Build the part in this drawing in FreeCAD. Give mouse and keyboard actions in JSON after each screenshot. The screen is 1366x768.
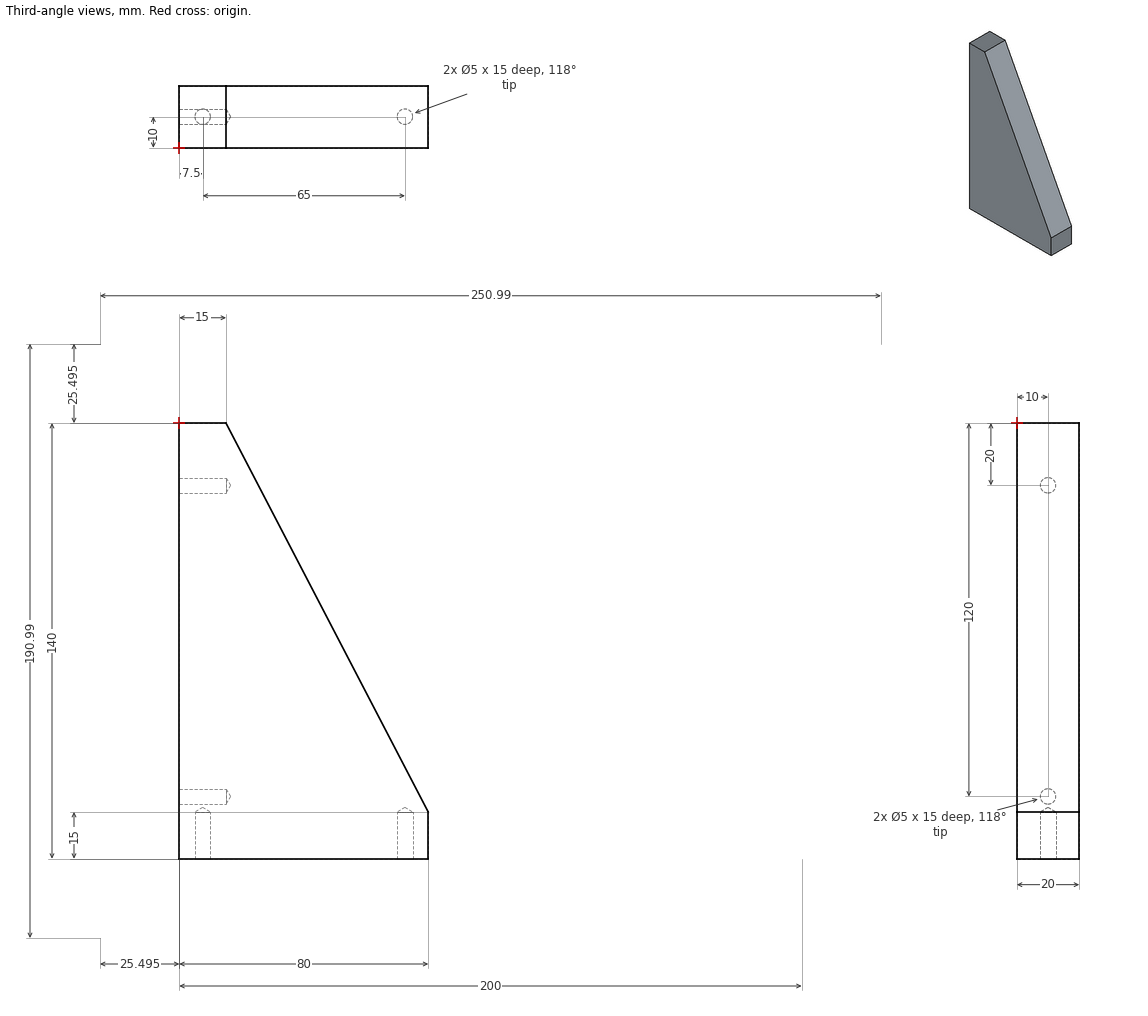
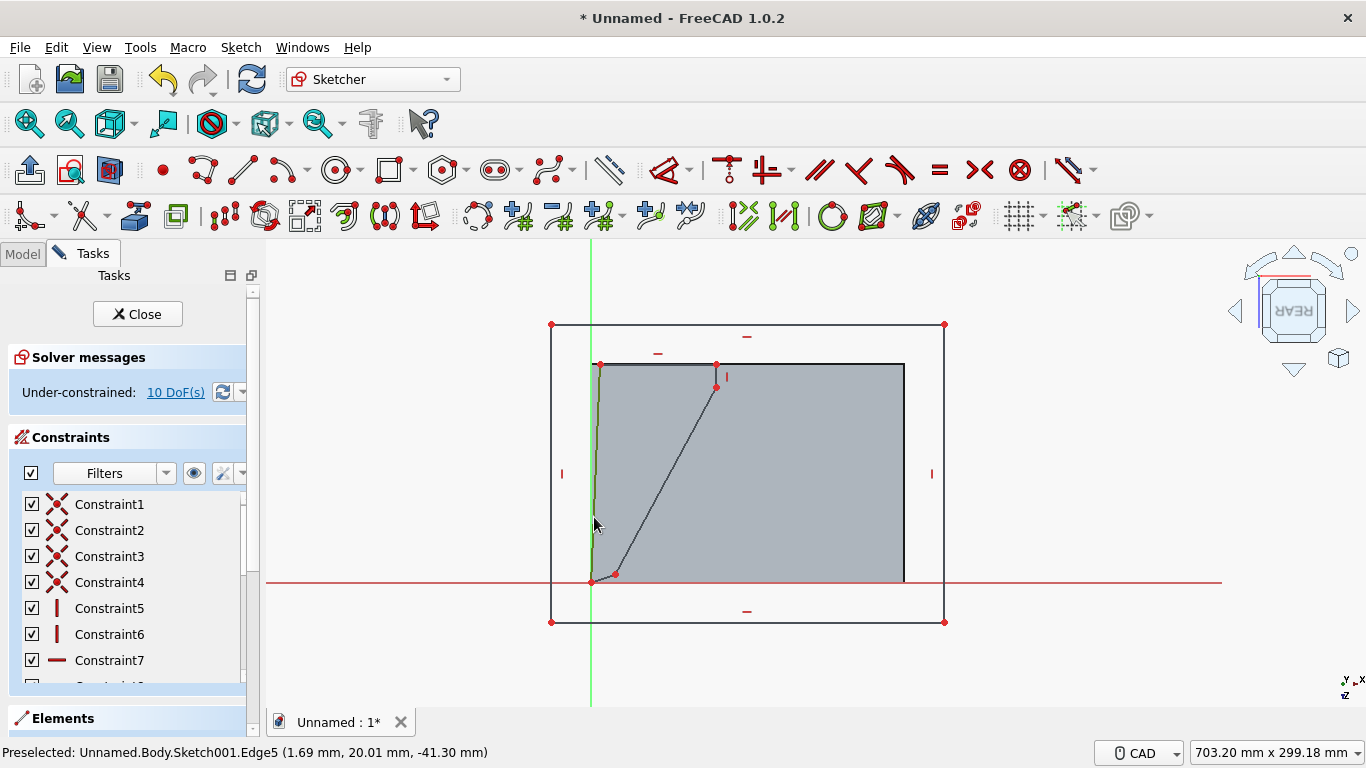
{"action": "left_click", "coordinate": [794, 170]}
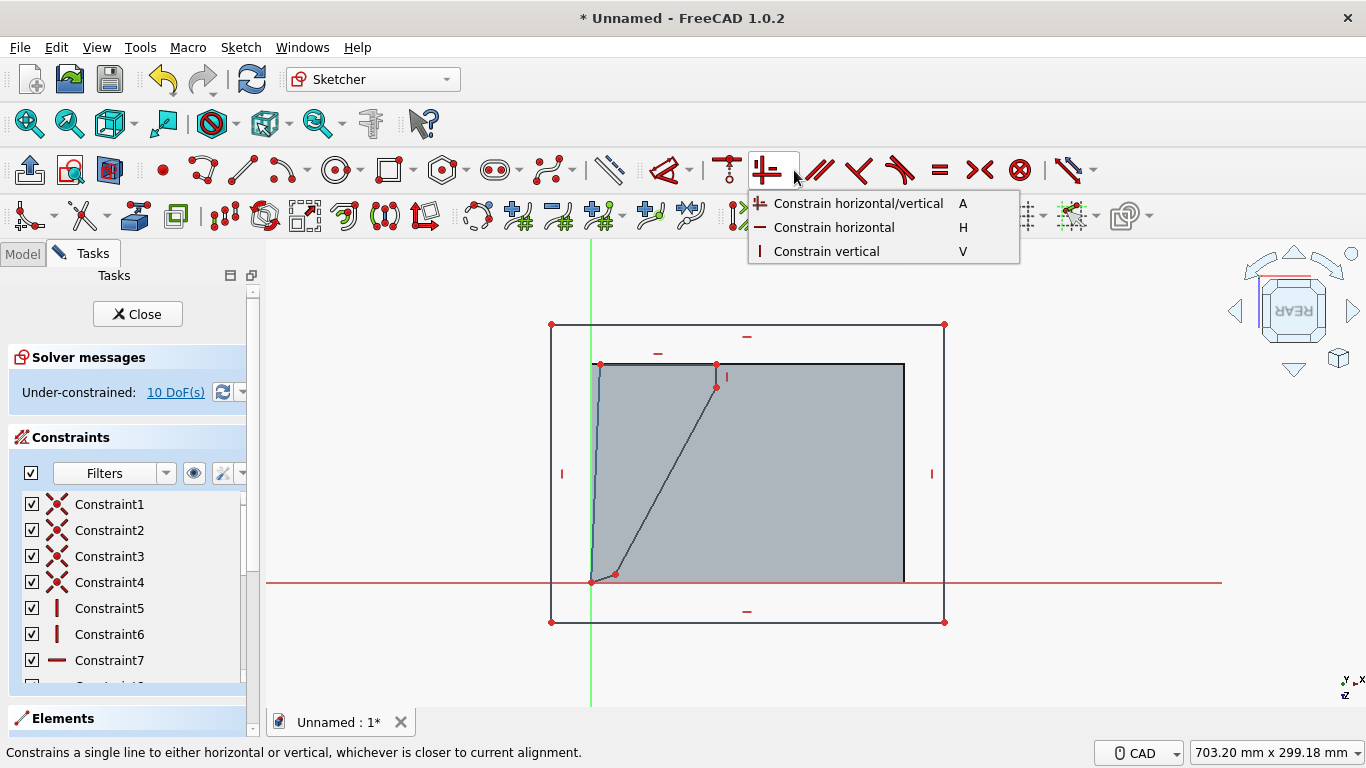
{"action": "left_click", "coordinate": [884, 251]}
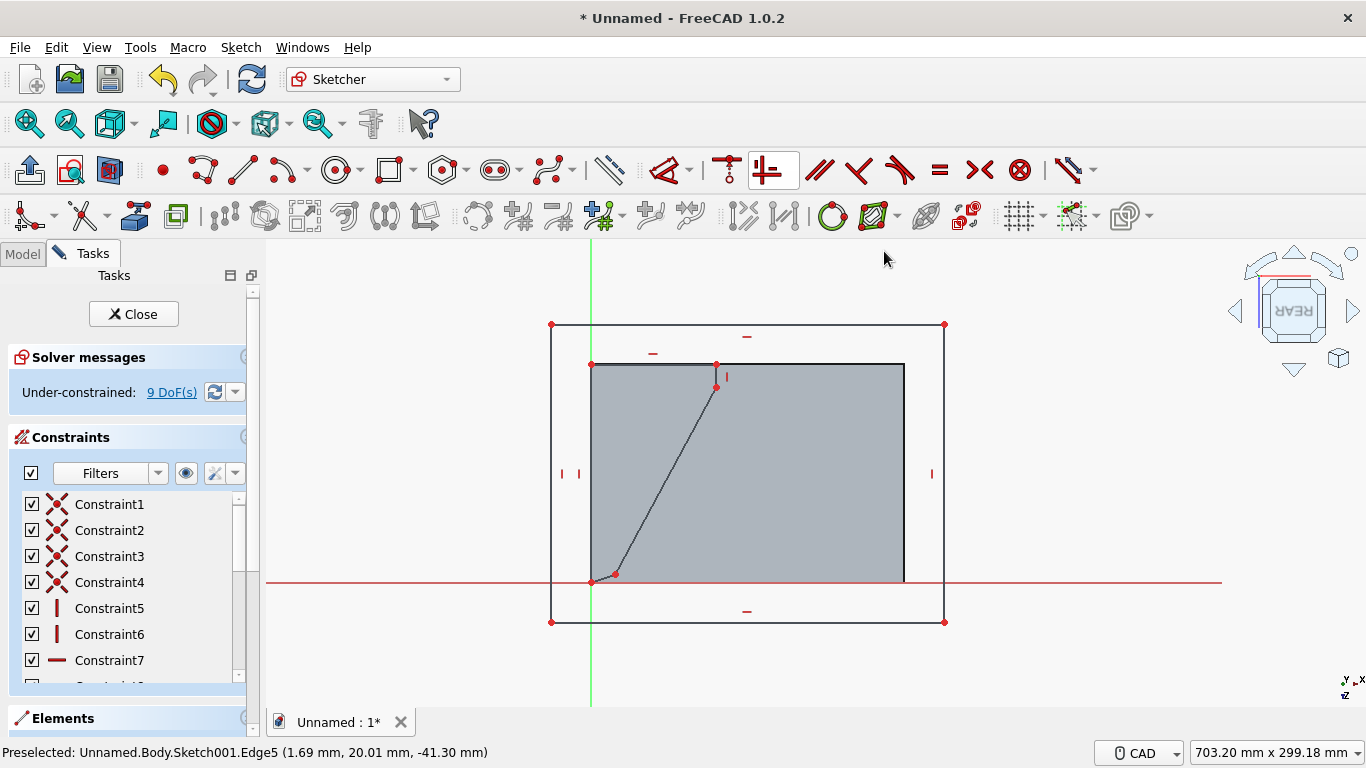
{"action": "scroll", "coordinate": [601, 580], "scroll_direction": "up", "scroll_amount": 2}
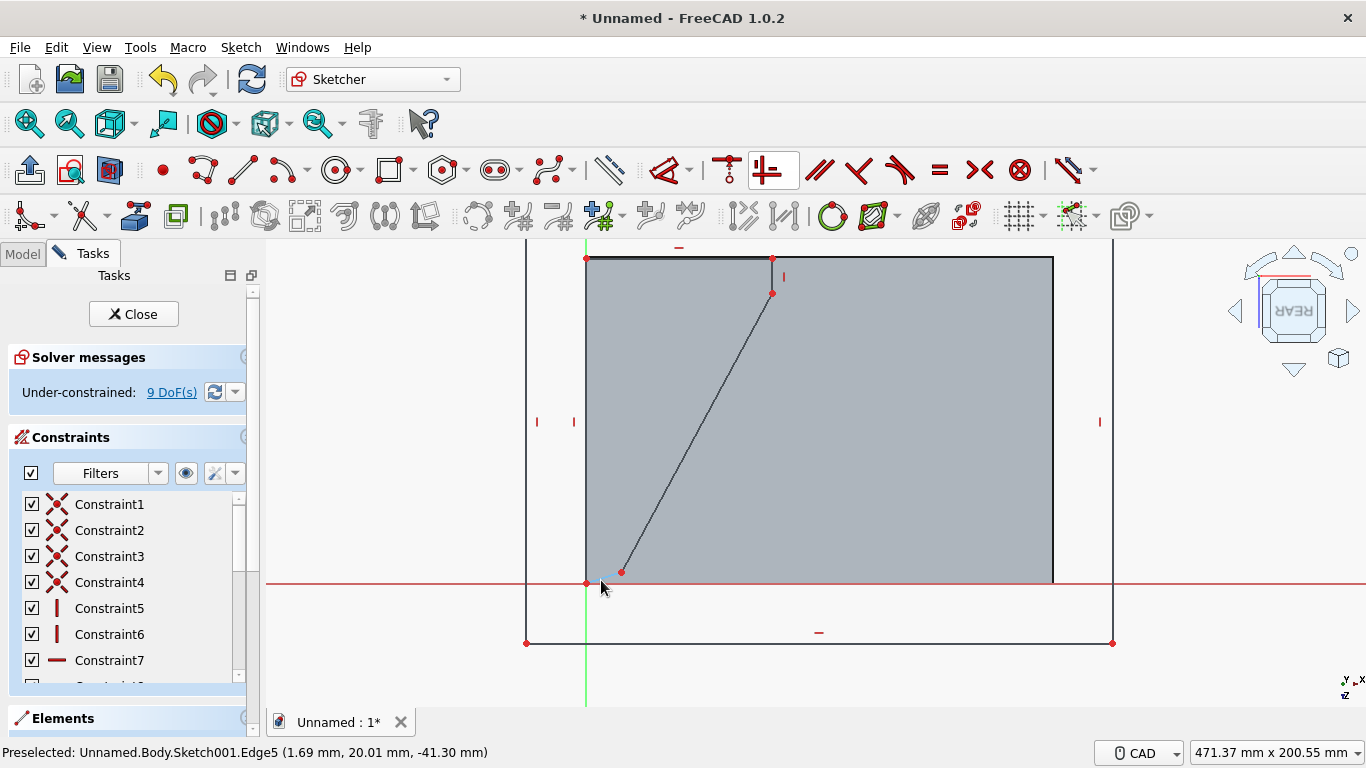
{"action": "left_click", "coordinate": [600, 579]}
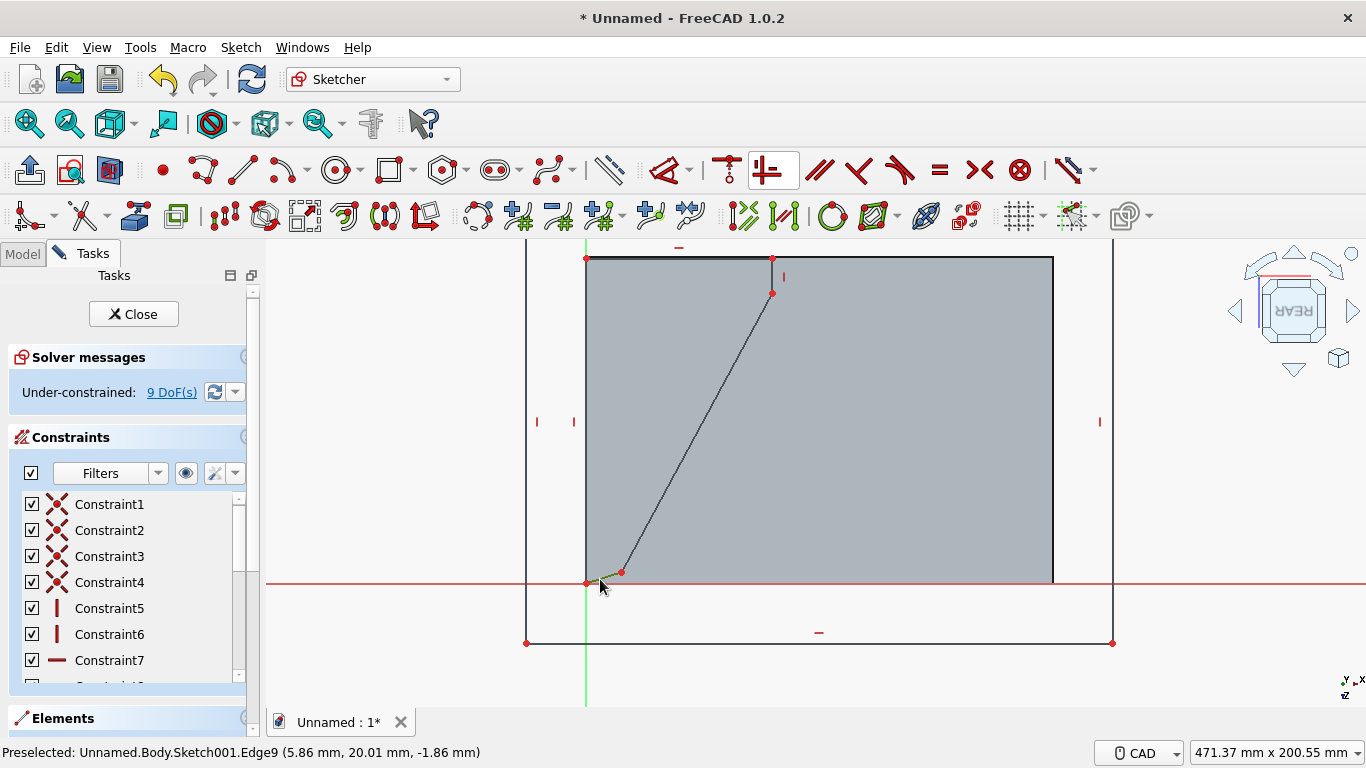
{"action": "key", "text": "h"}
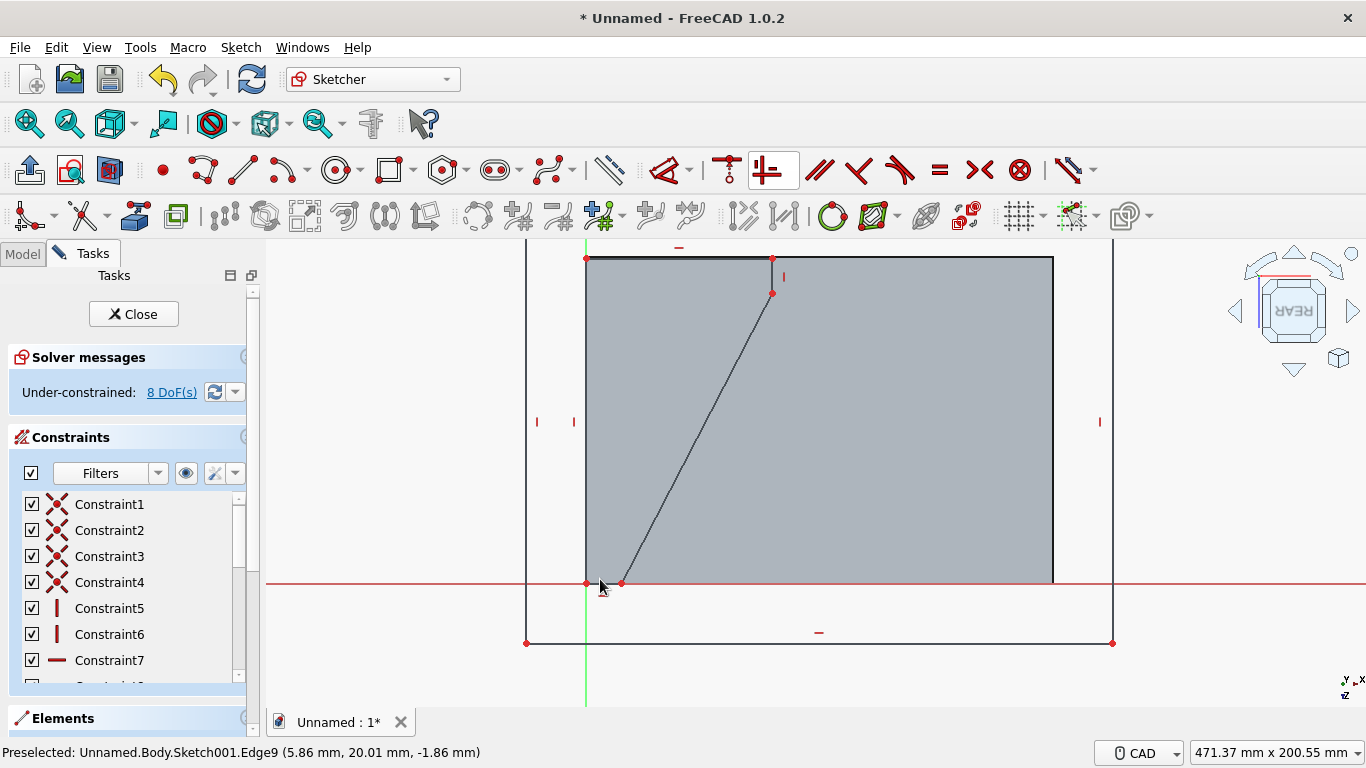
{"action": "key", "text": "d"}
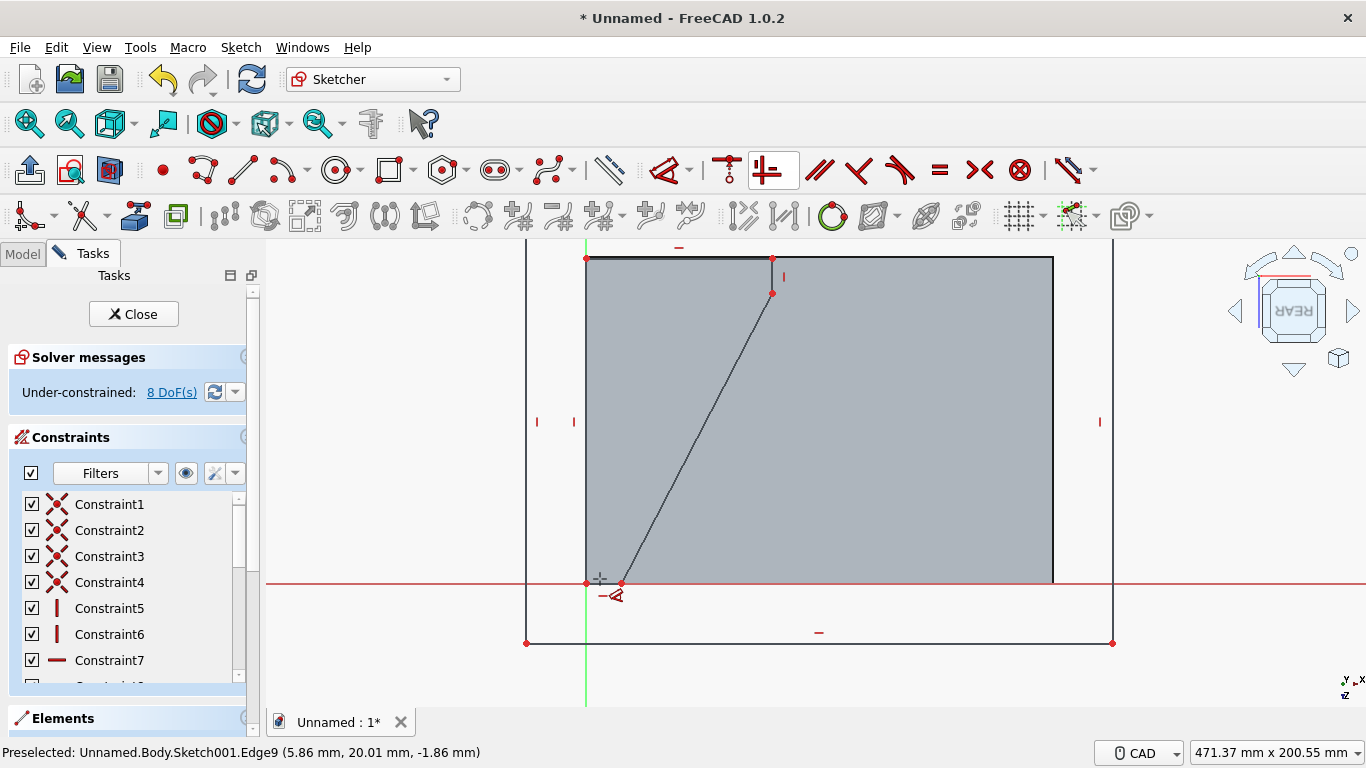
{"action": "scroll", "coordinate": [601, 580], "scroll_direction": "down", "scroll_amount": 2}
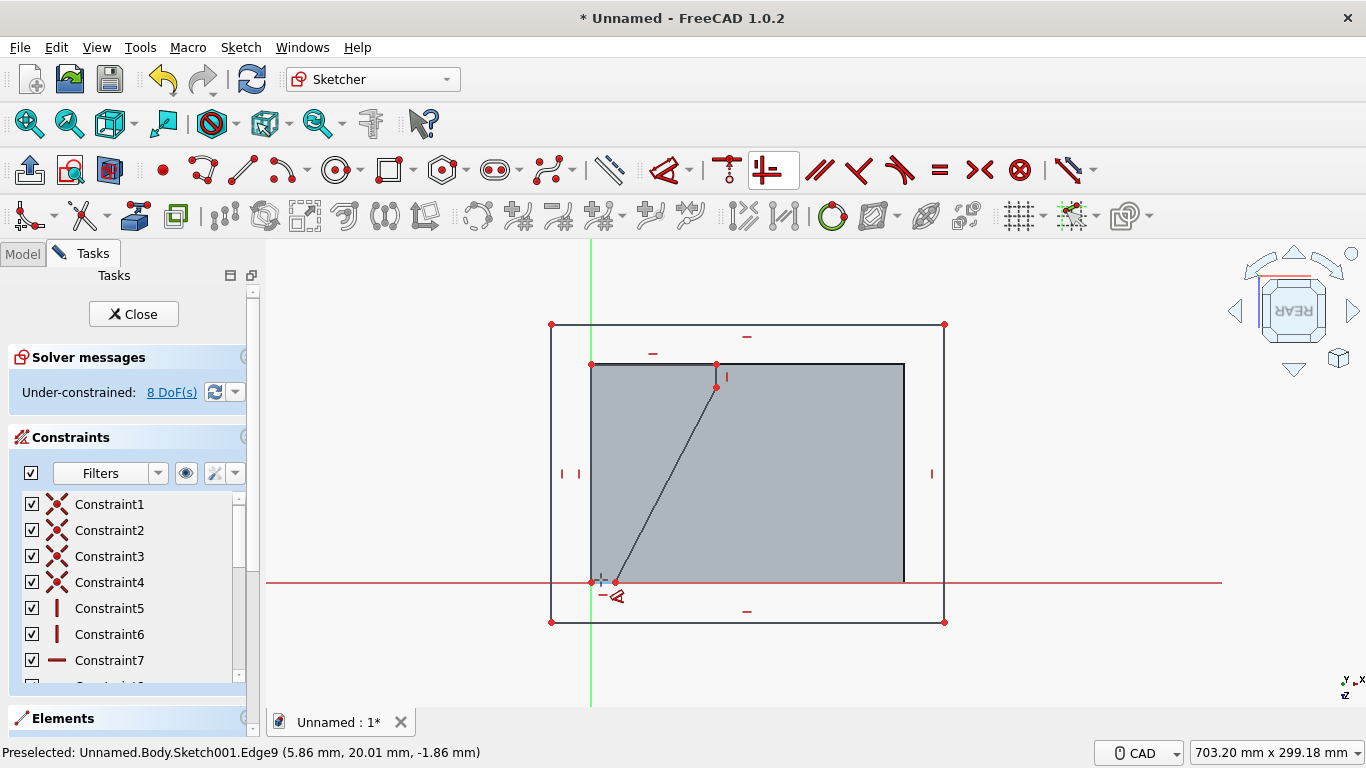
{"action": "left_click", "coordinate": [629, 365]}
{"action": "left_click", "coordinate": [654, 399]}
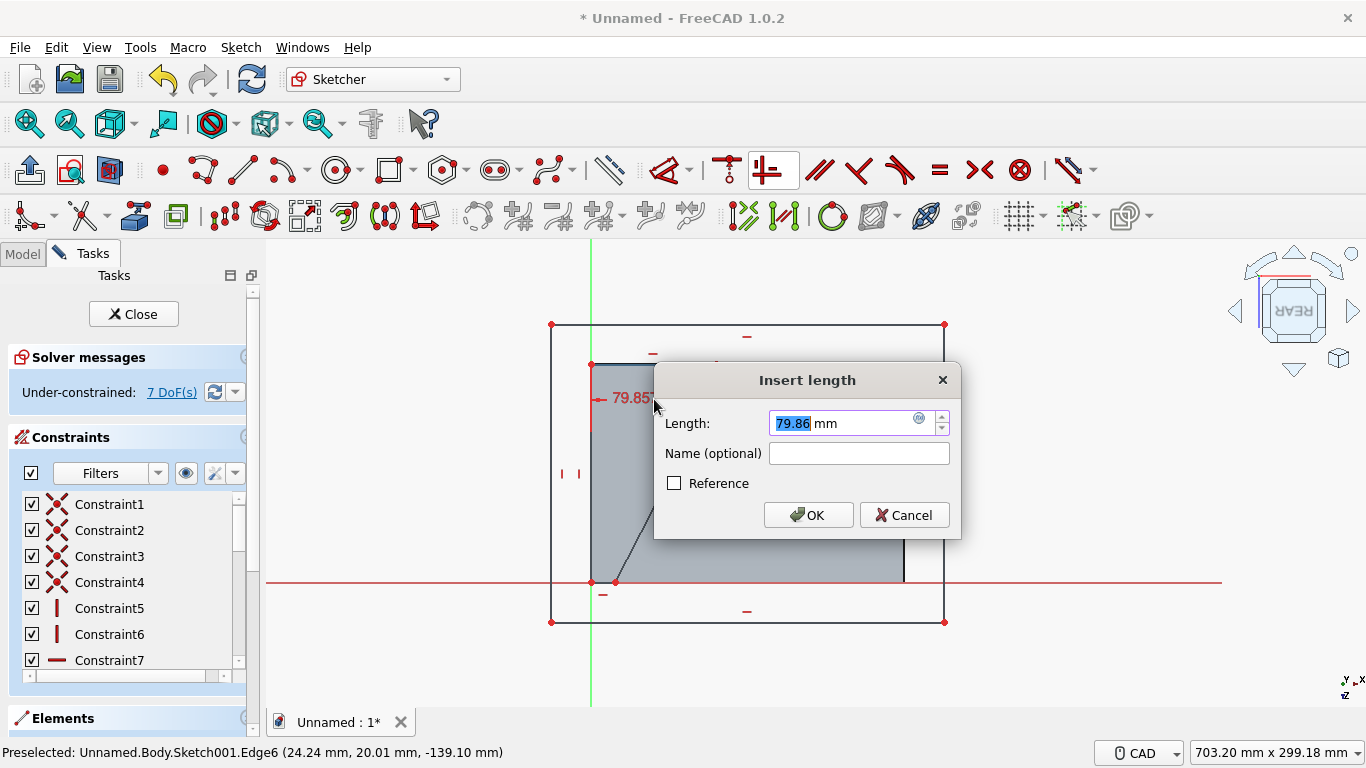
{"action": "type", "text": "80"}
{"action": "key", "text": "Return"}